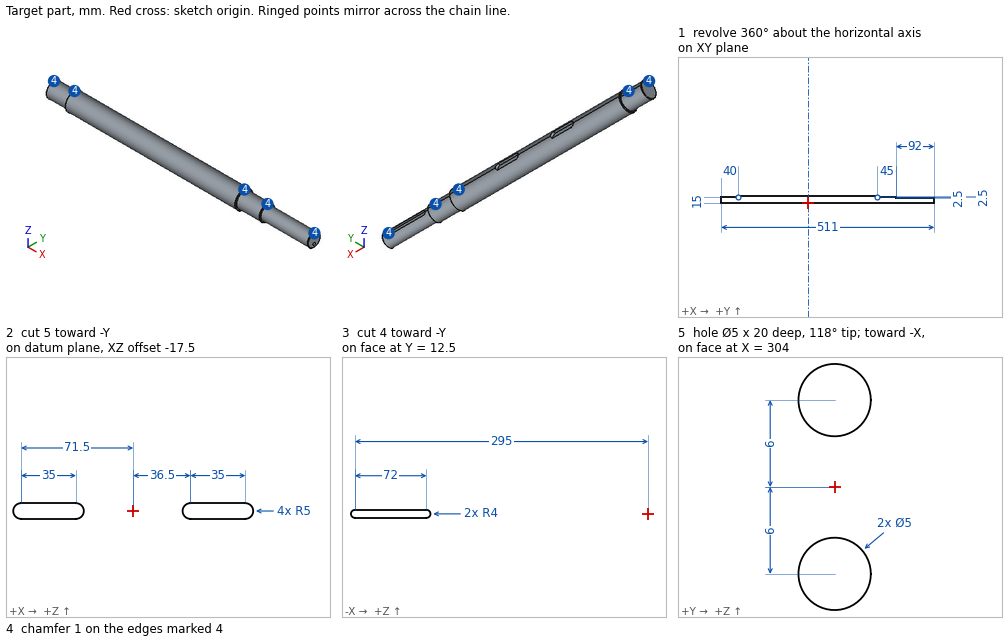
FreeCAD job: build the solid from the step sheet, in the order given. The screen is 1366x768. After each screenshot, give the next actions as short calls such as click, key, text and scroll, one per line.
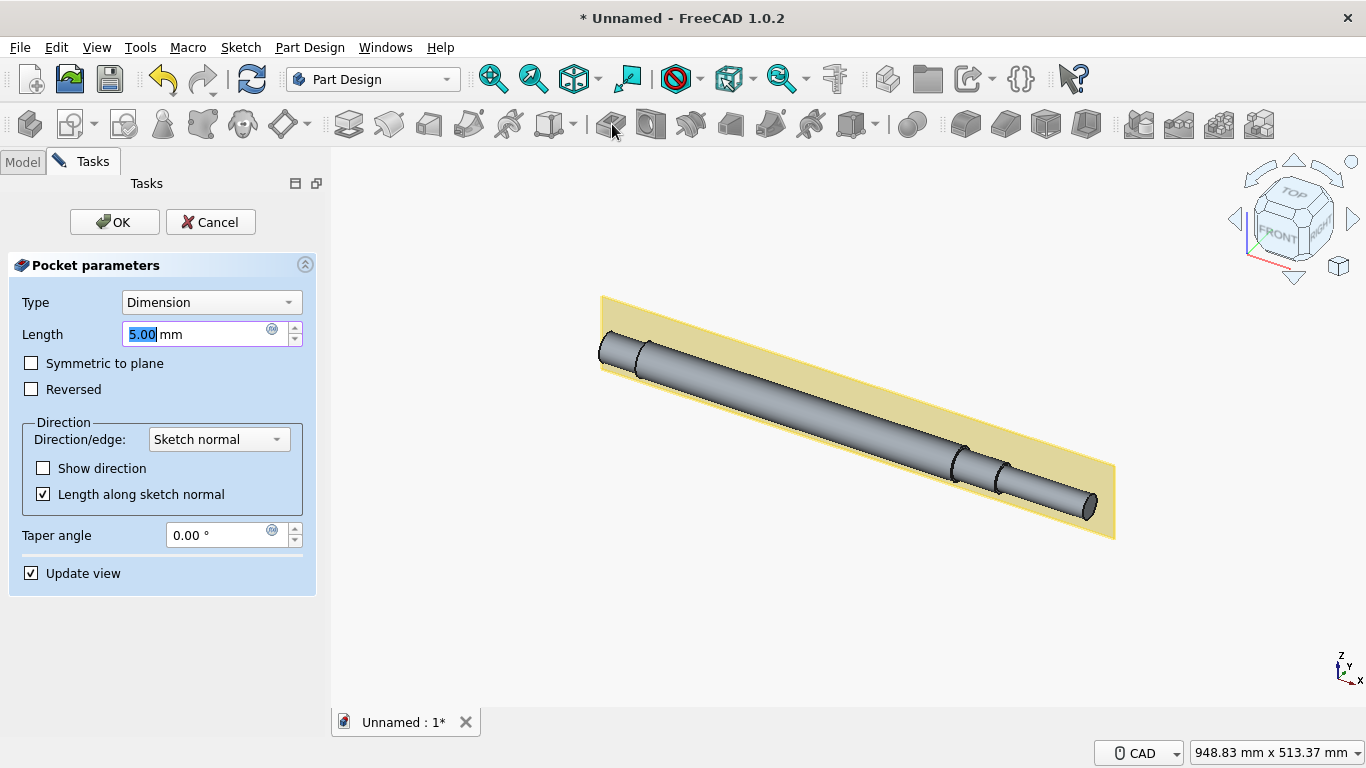
text(5)
key(Tab)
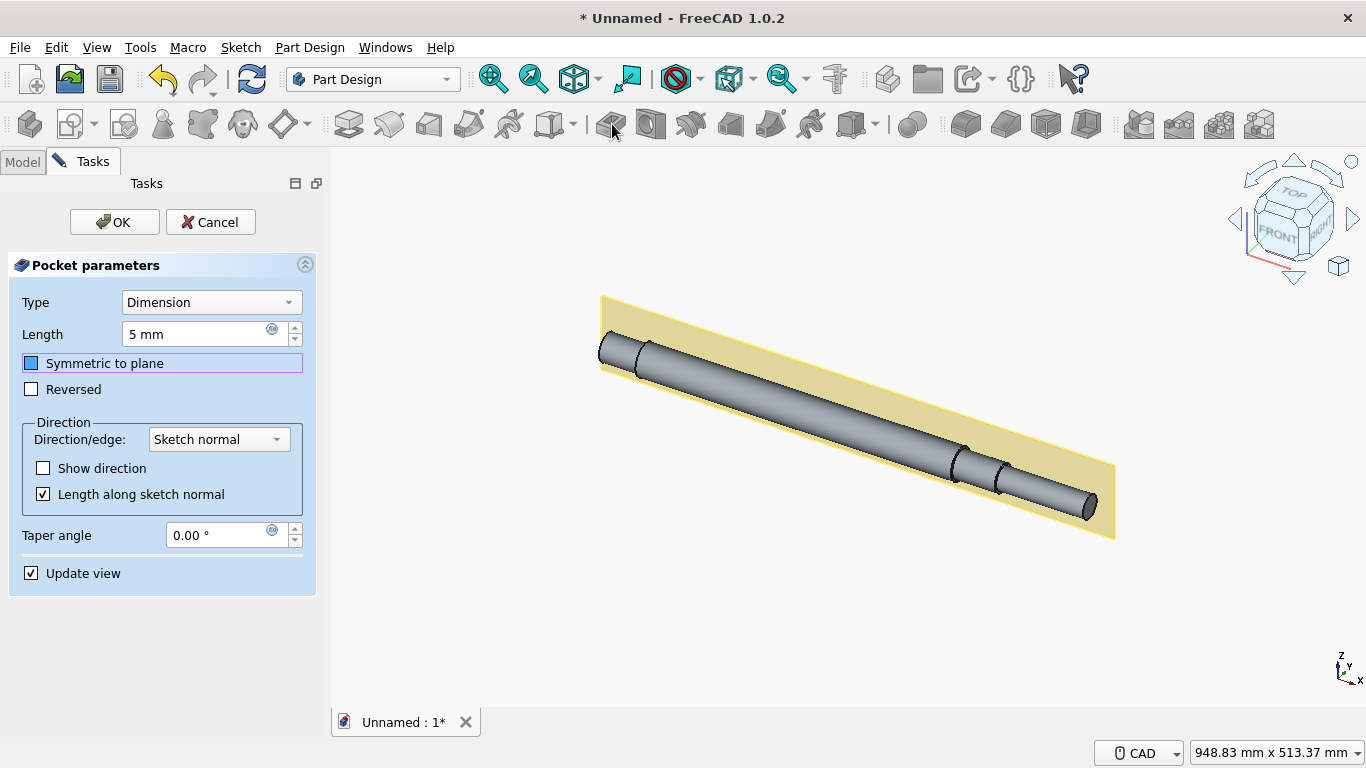
click(30, 389)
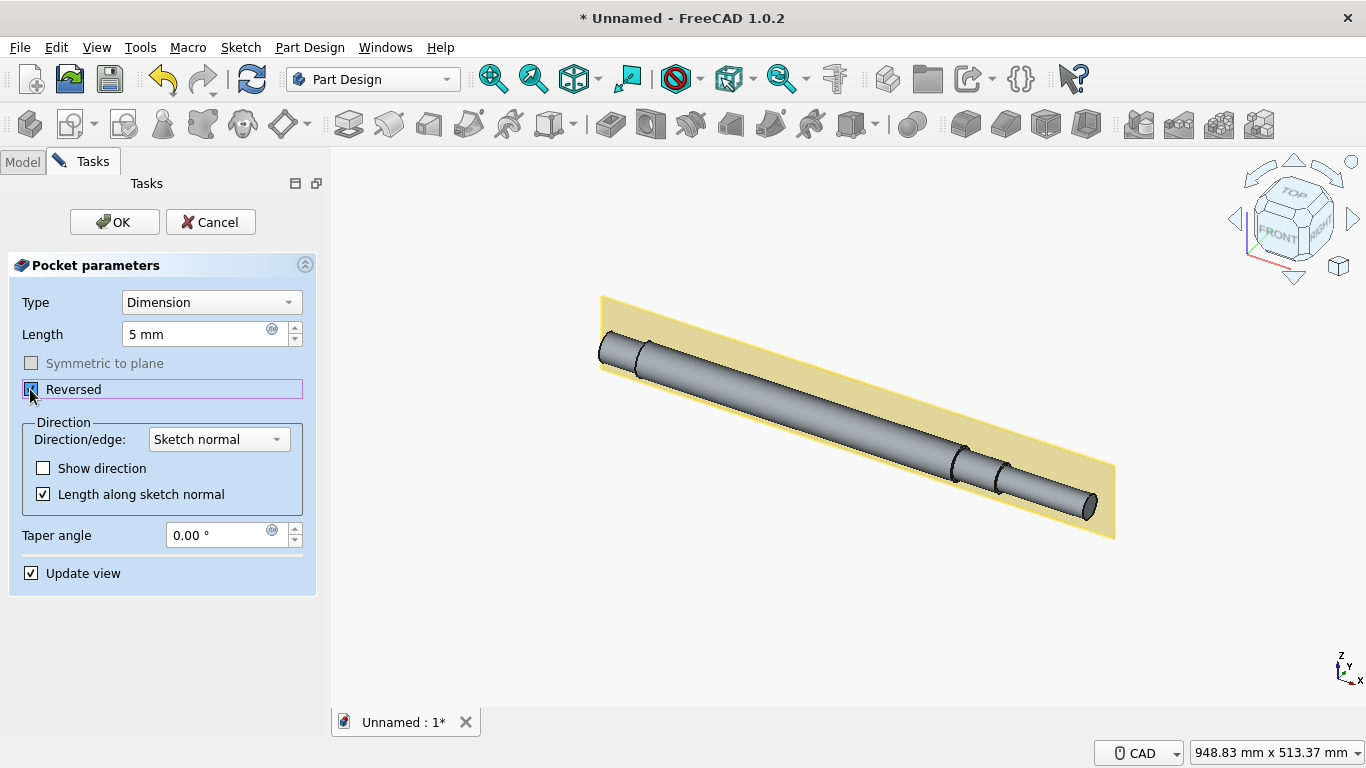
click(115, 222)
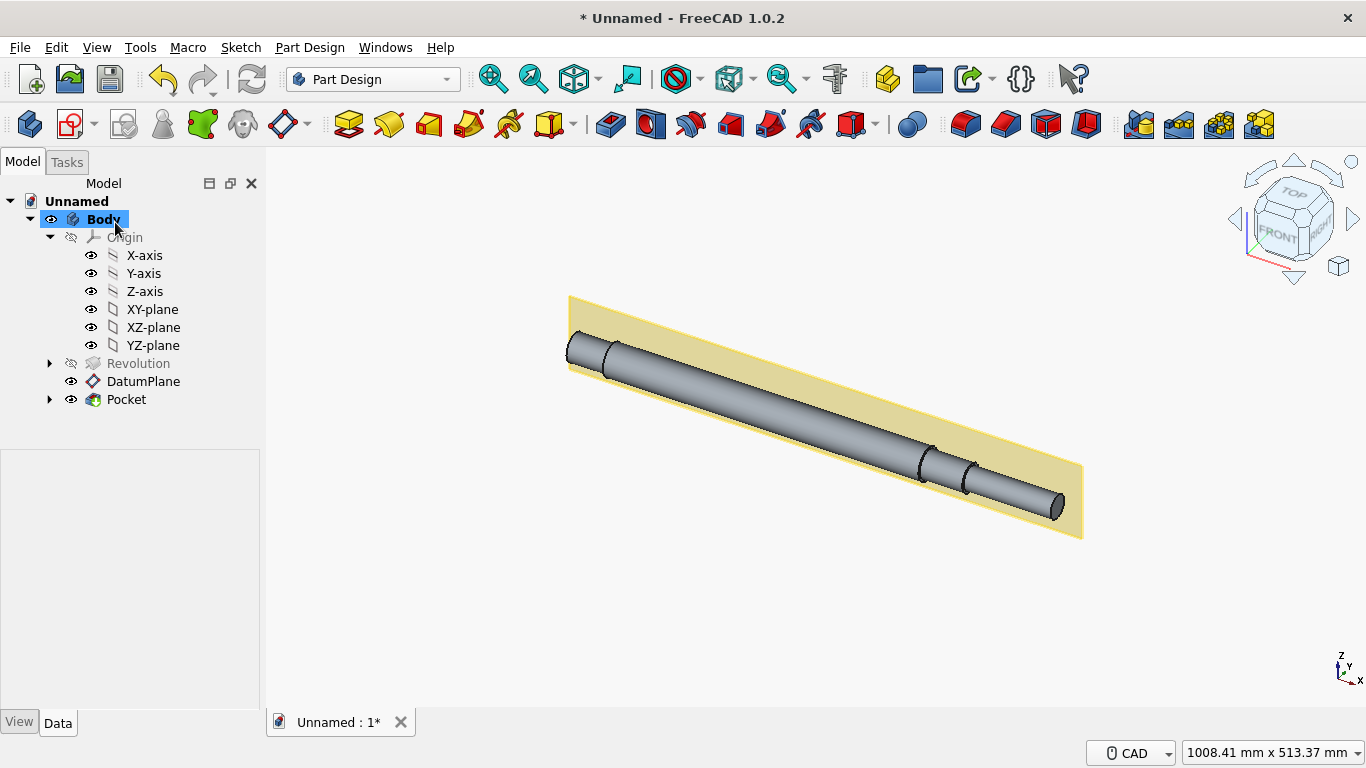
click(116, 381)
key(space)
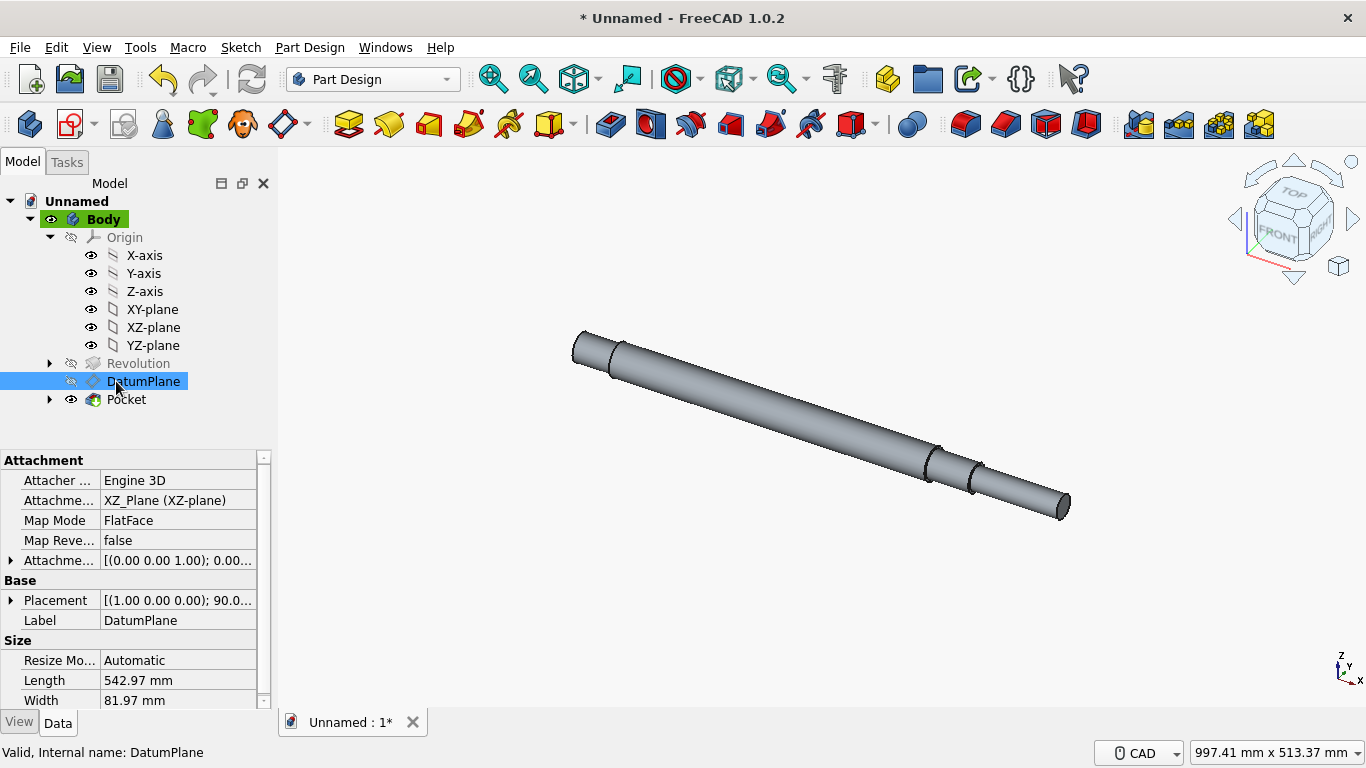
key(4)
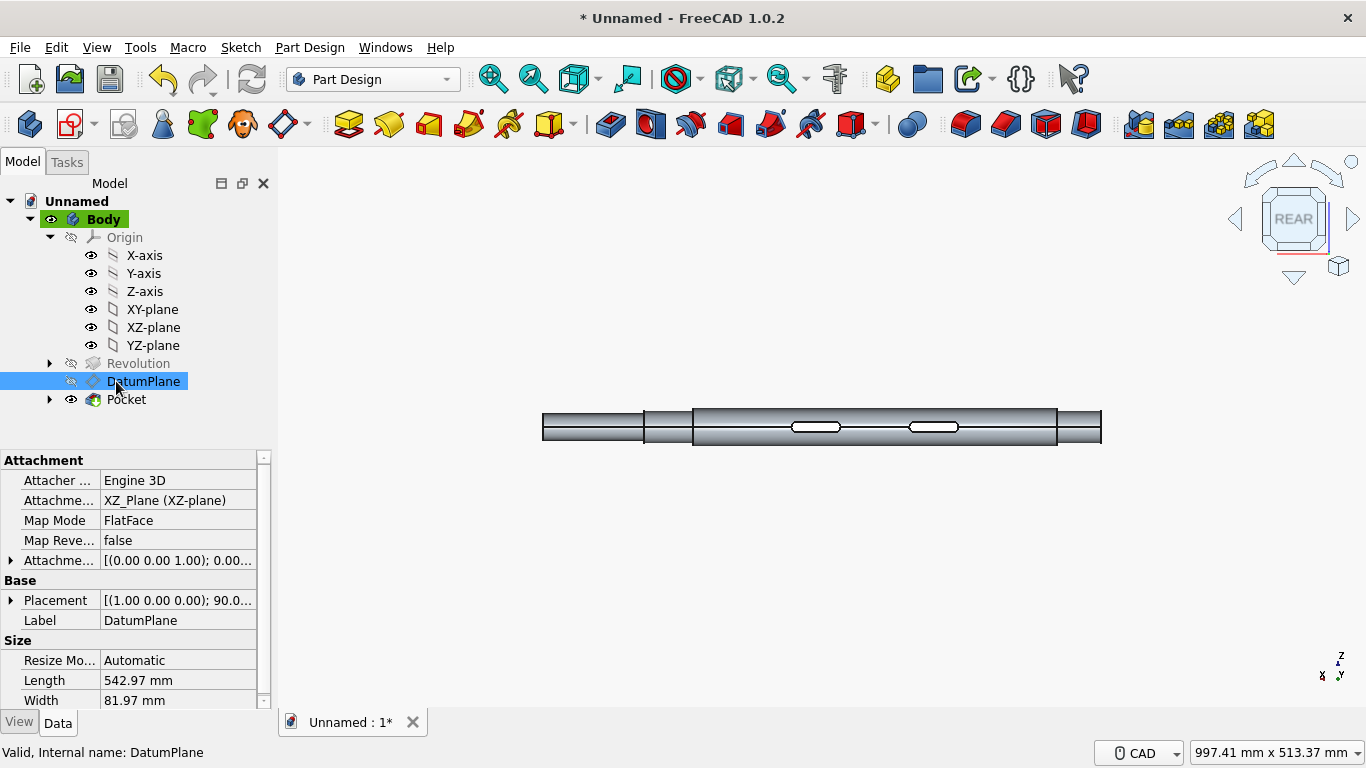
scroll(802, 426, up, 4)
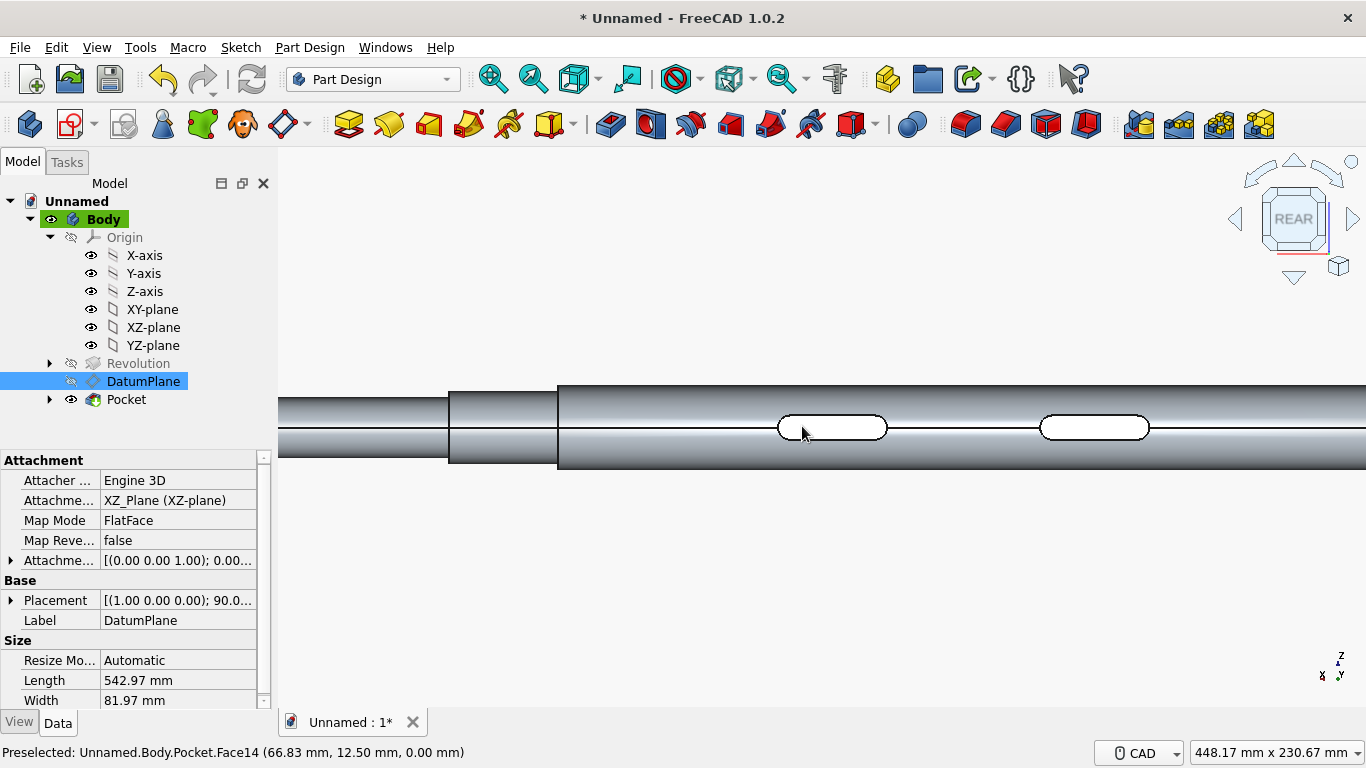
click(801, 427)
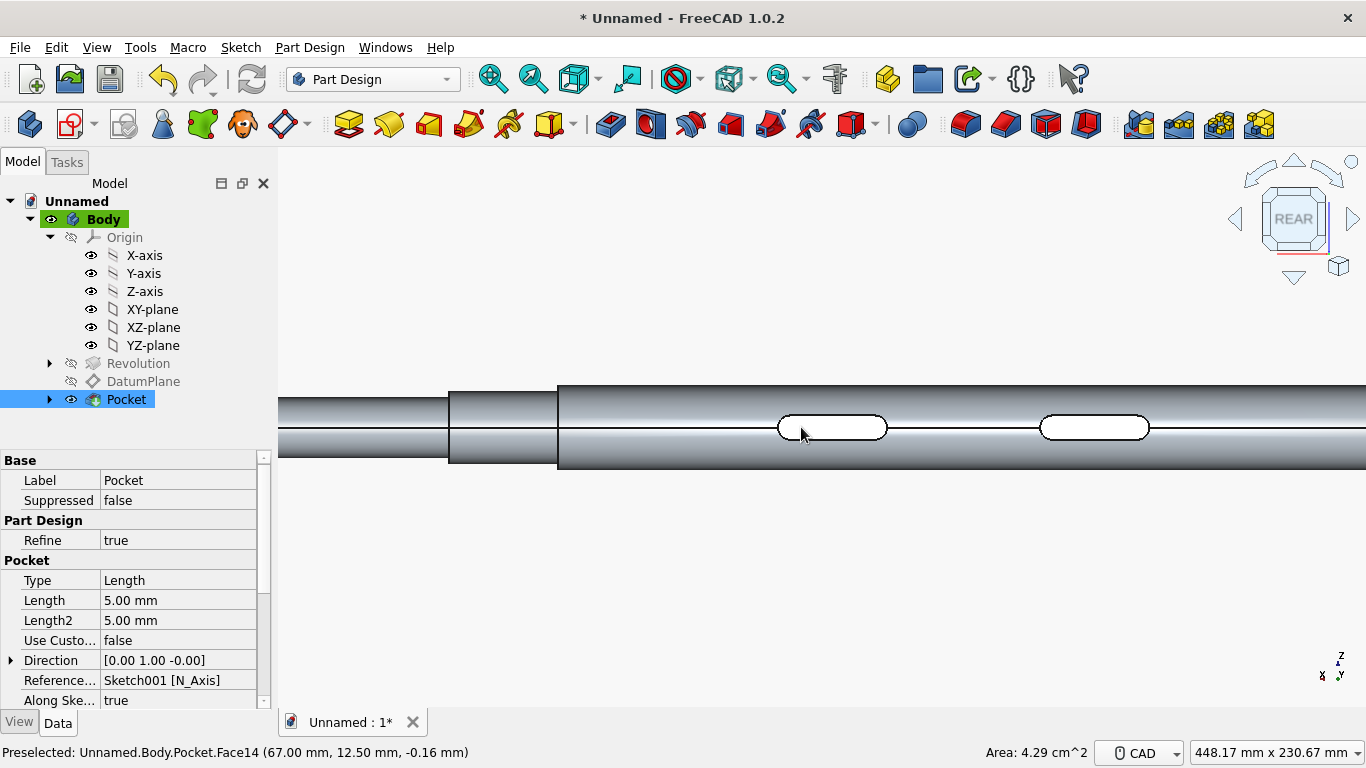
click(70, 124)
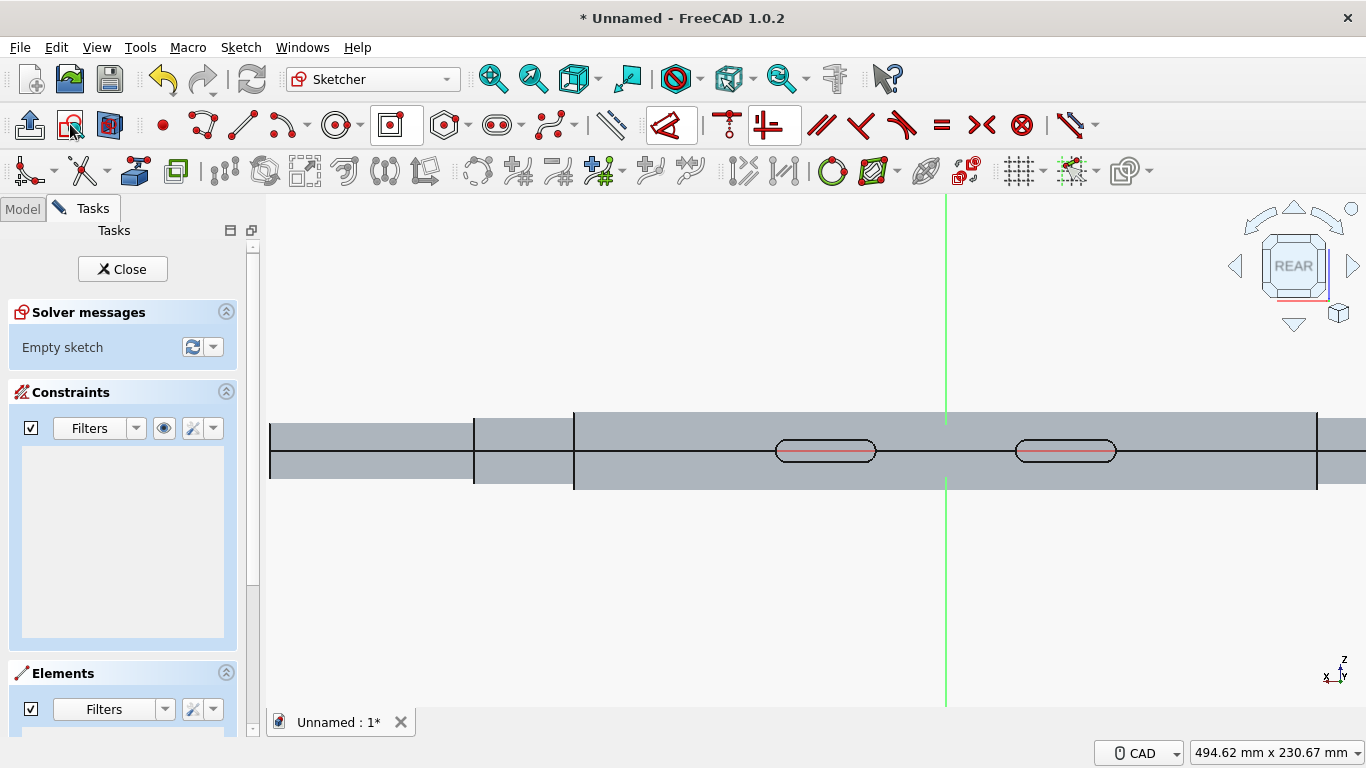
click(110, 126)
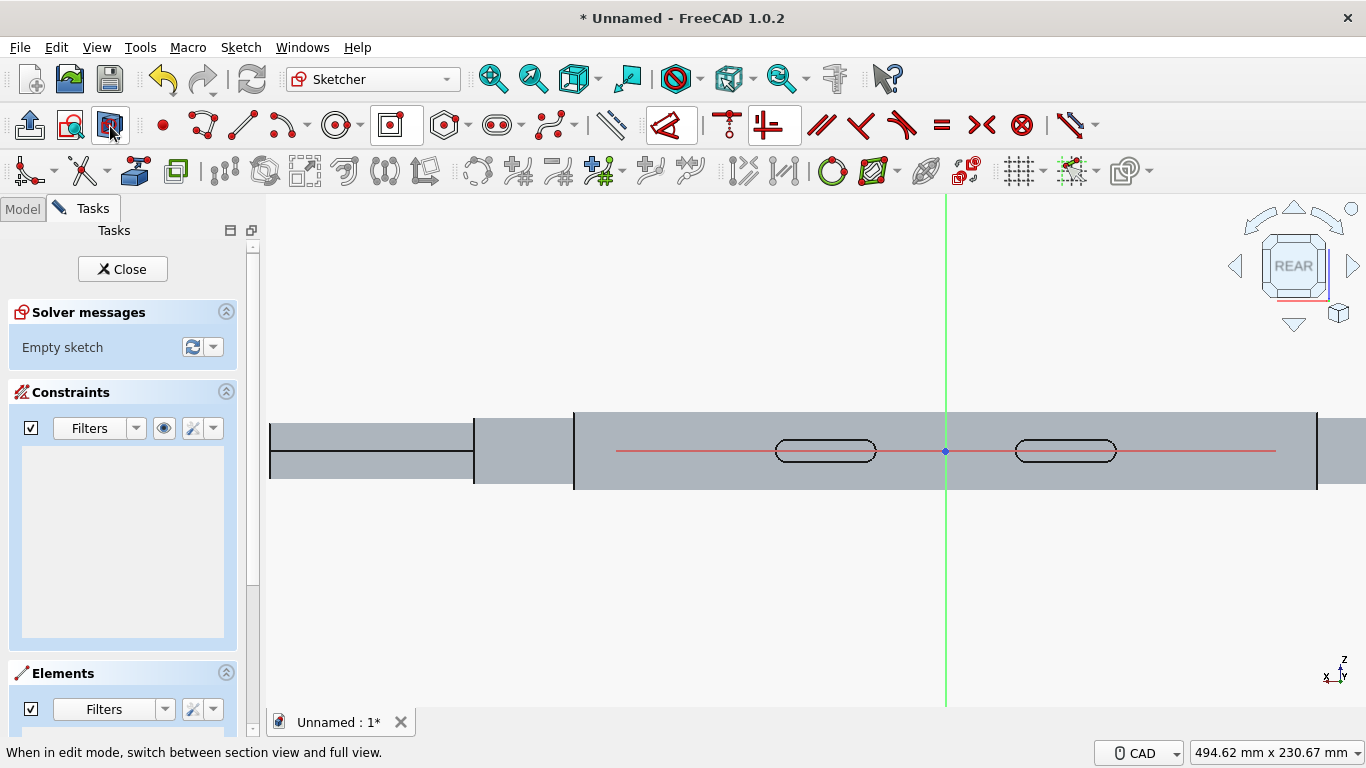
scroll(748, 450, down, 5)